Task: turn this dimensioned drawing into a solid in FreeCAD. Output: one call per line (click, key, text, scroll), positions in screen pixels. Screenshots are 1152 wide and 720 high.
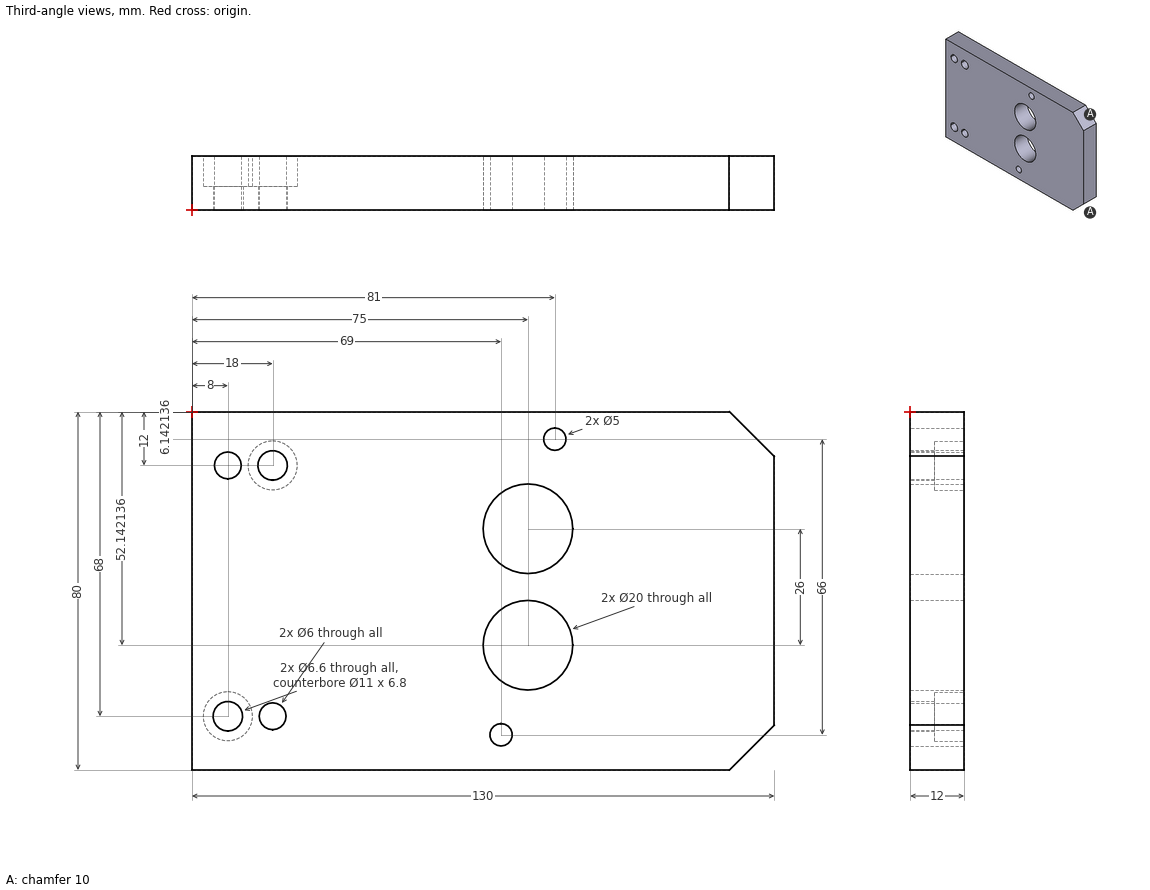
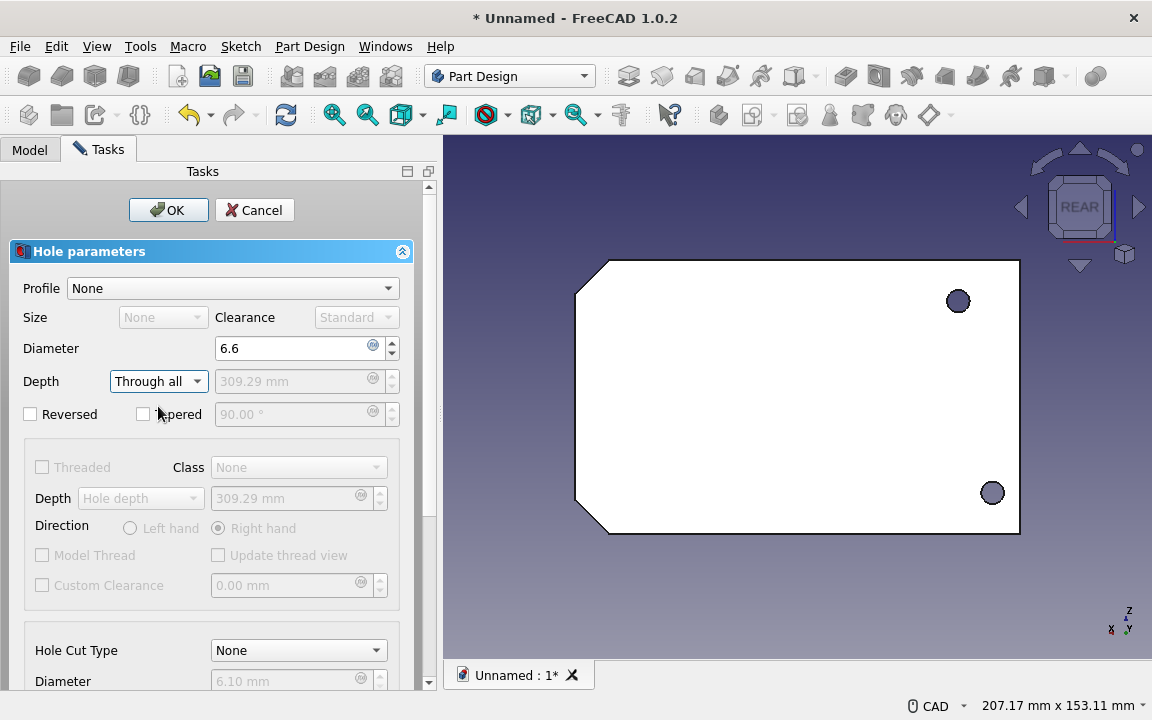
click(300, 650)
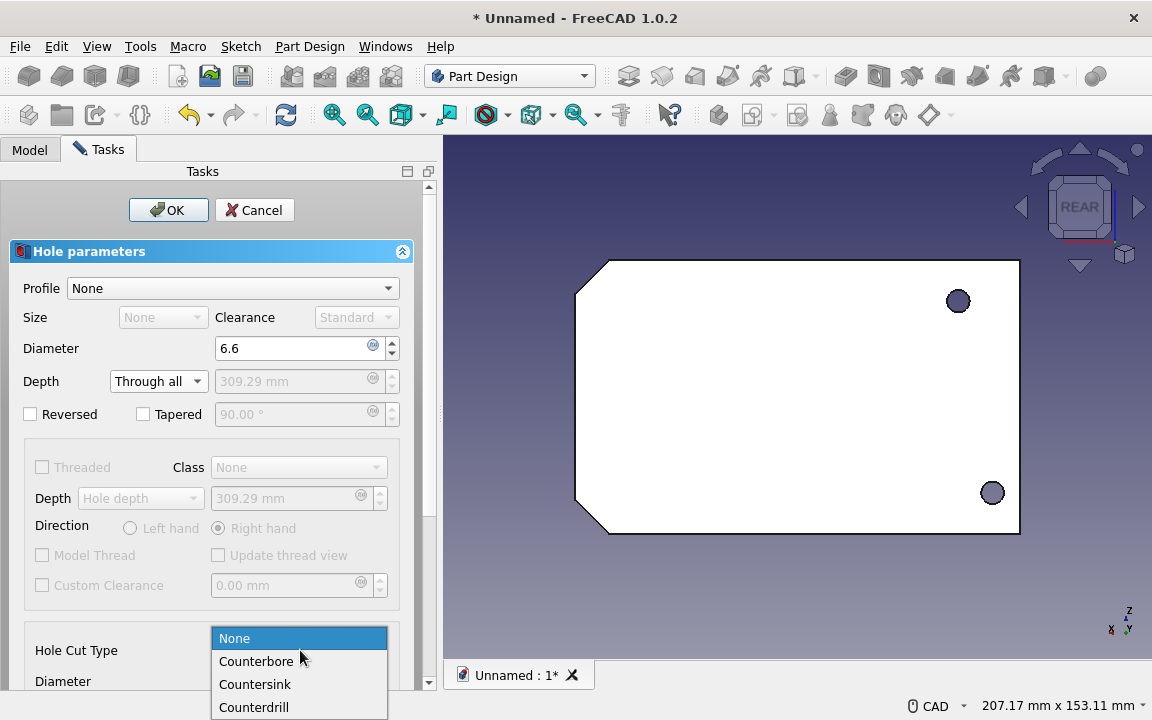
click(298, 662)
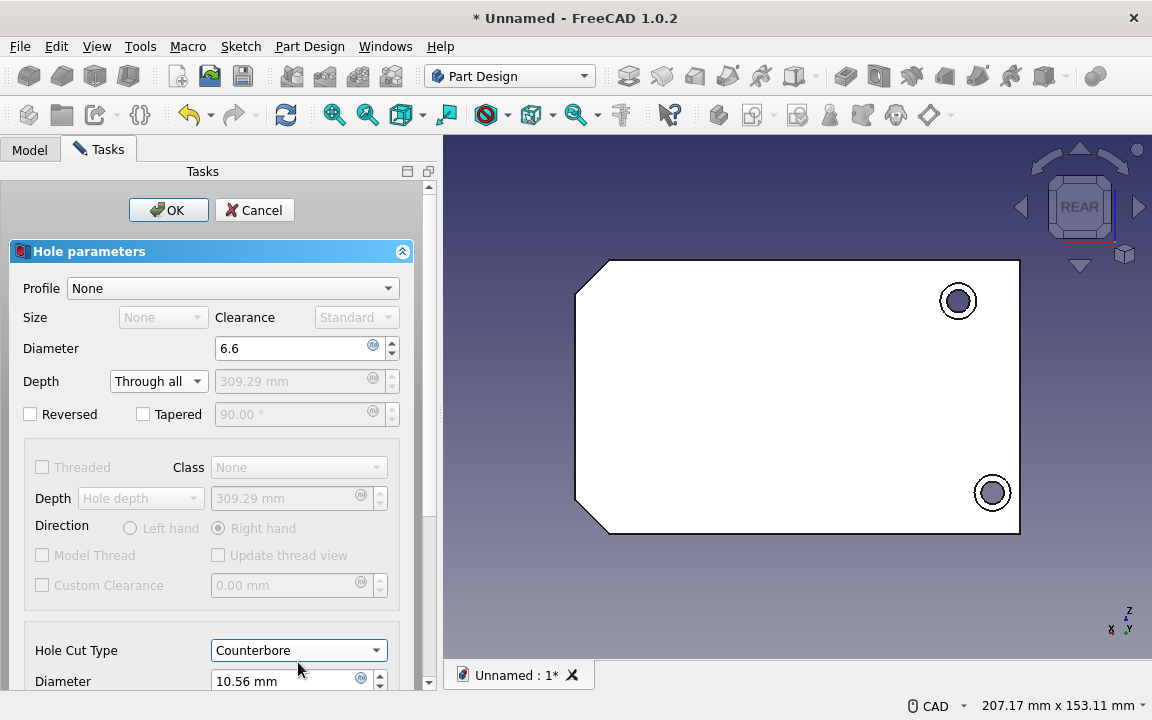
scroll(429, 436, down, 2)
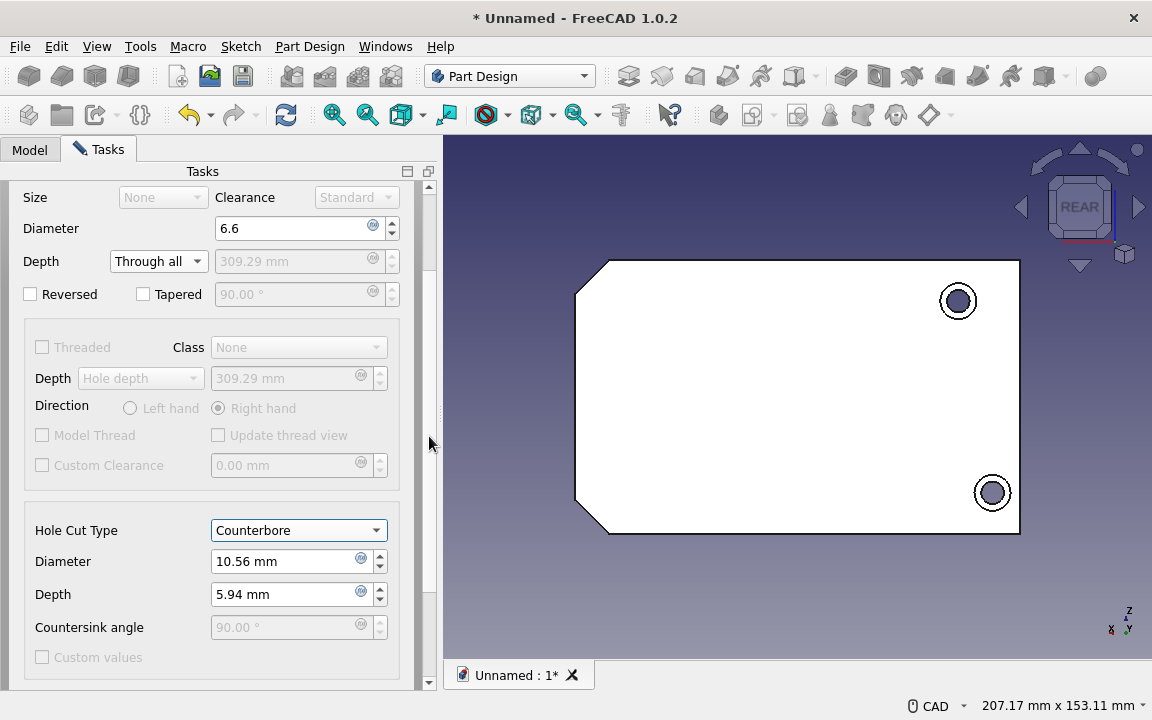
triple_click(292, 562)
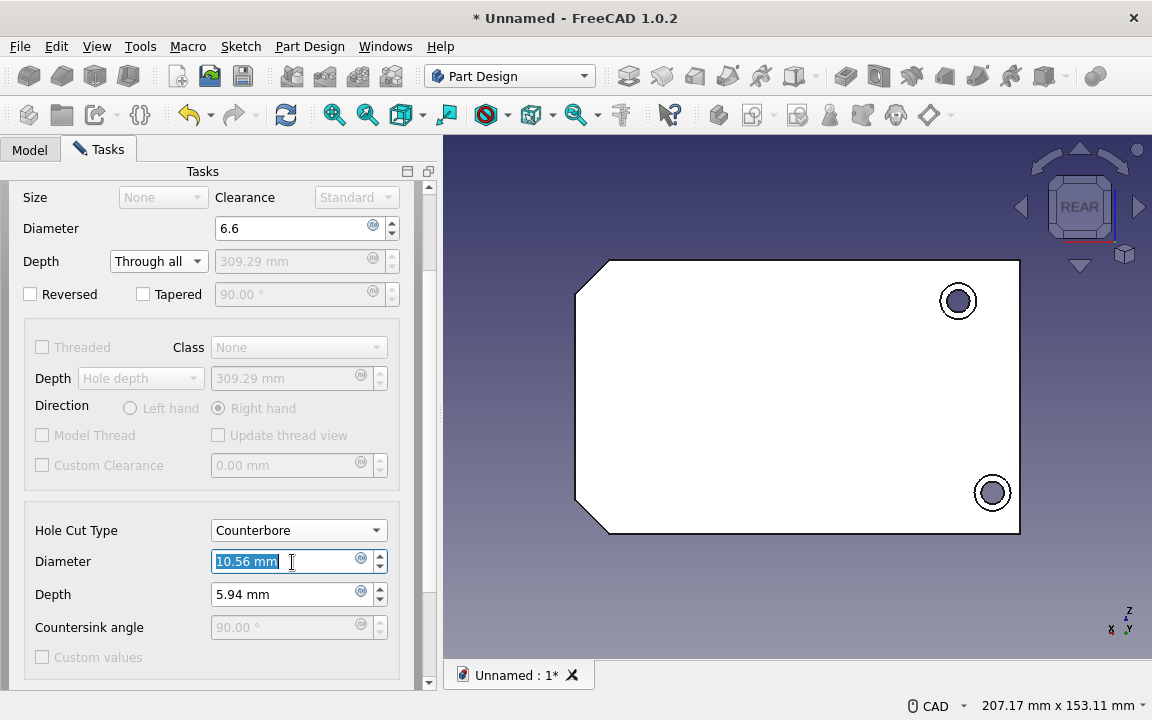
text(11)
key(Tab)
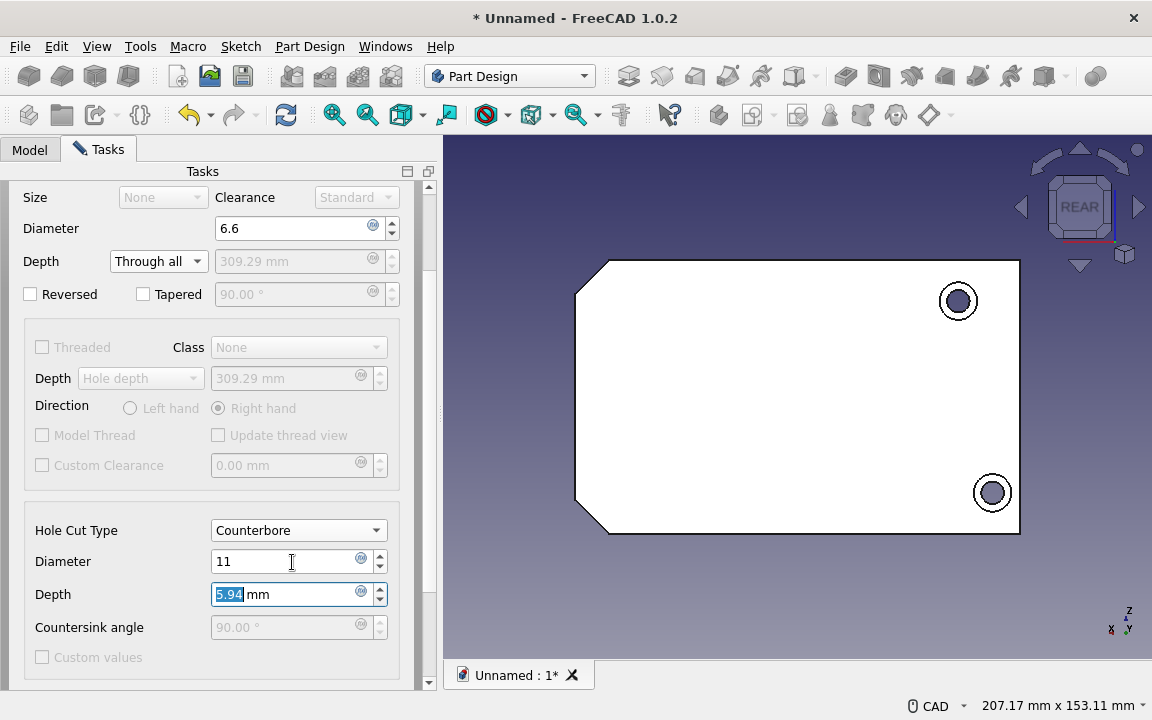
text(6.8)
key(Tab)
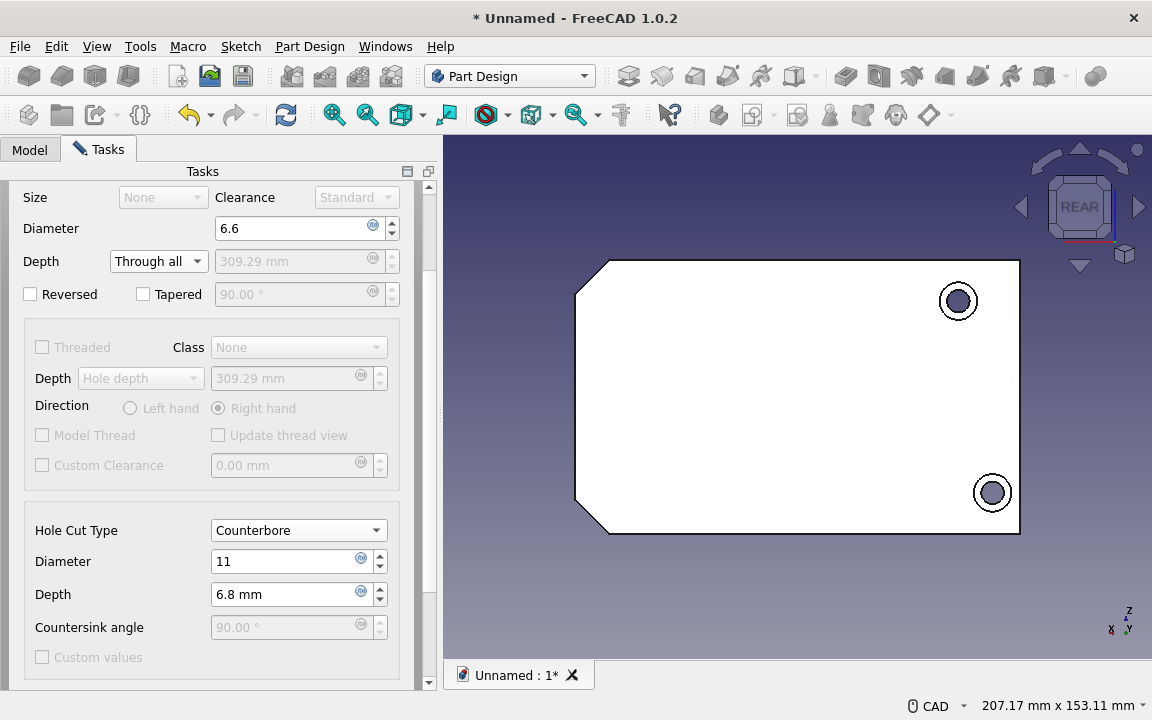
scroll(429, 436, up, 3)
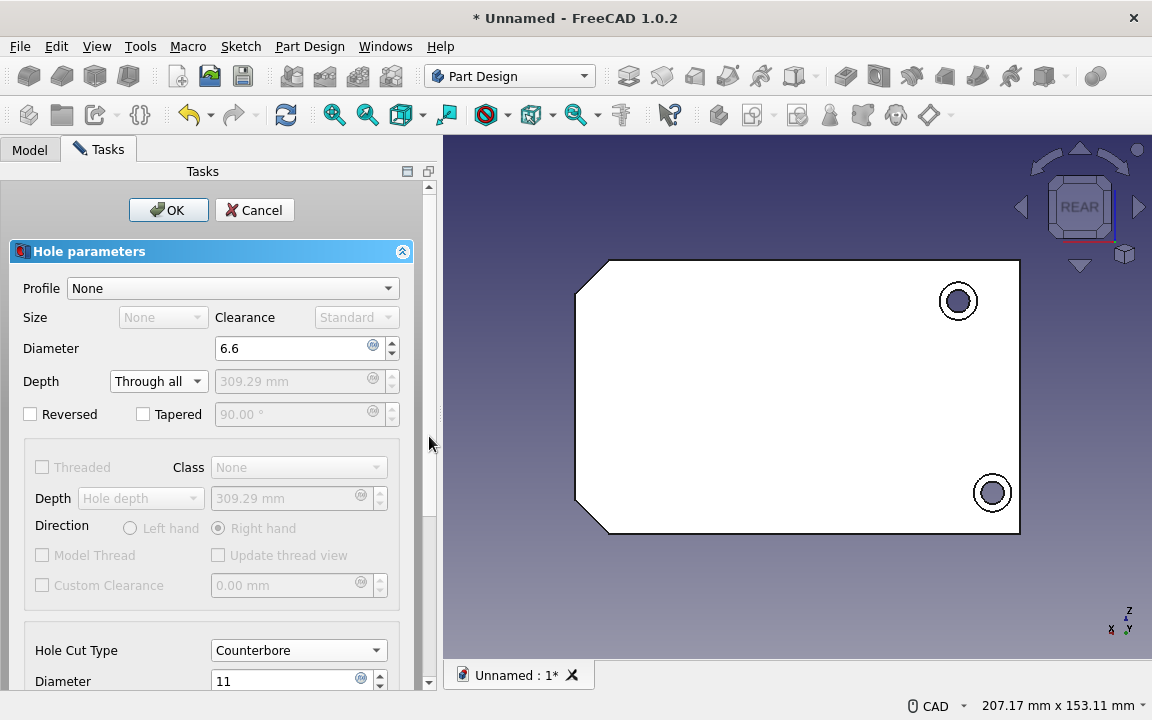
click(169, 210)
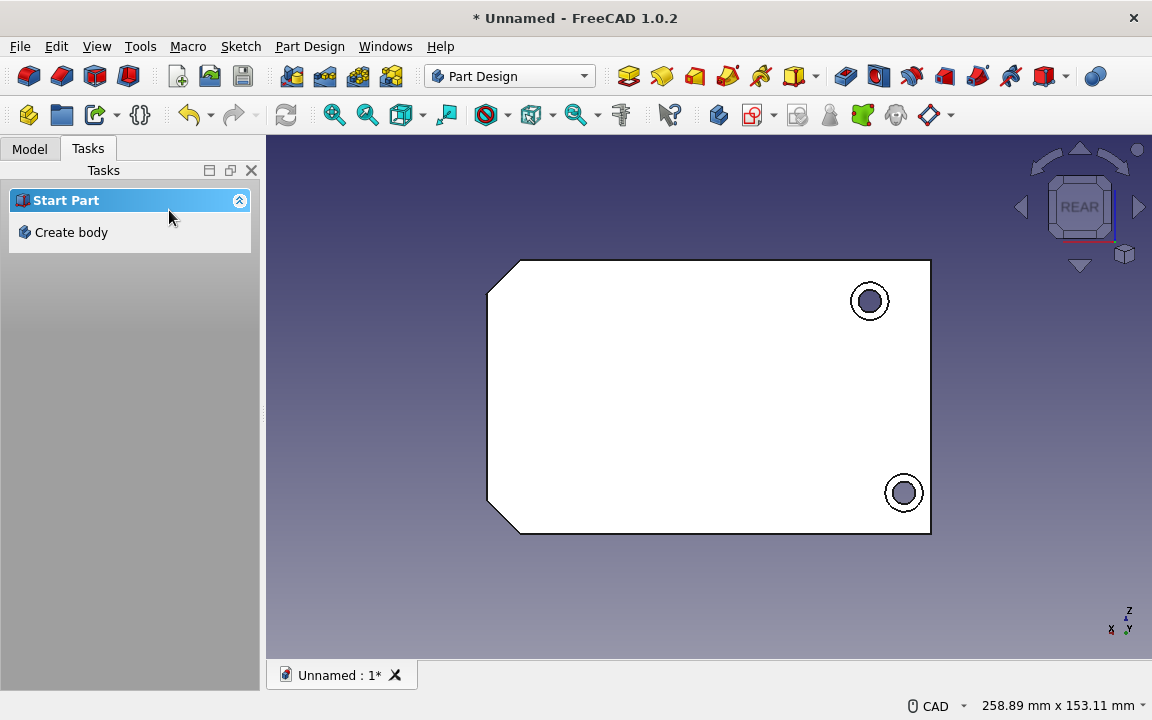
click(645, 396)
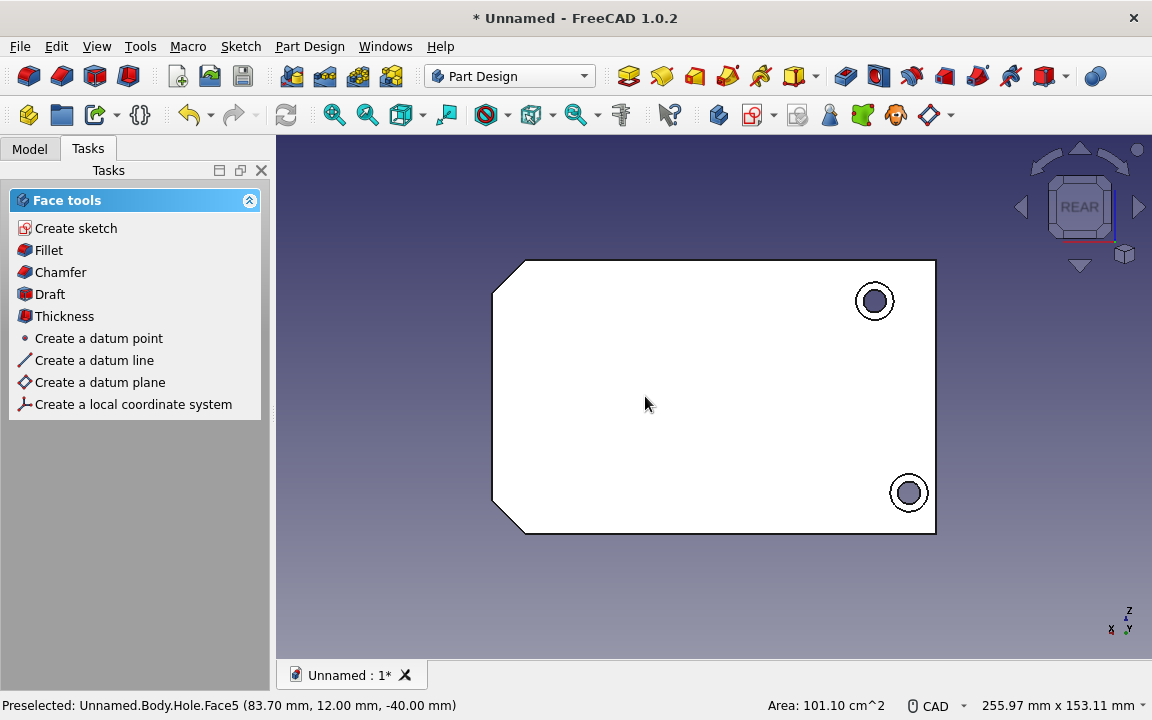
click(752, 116)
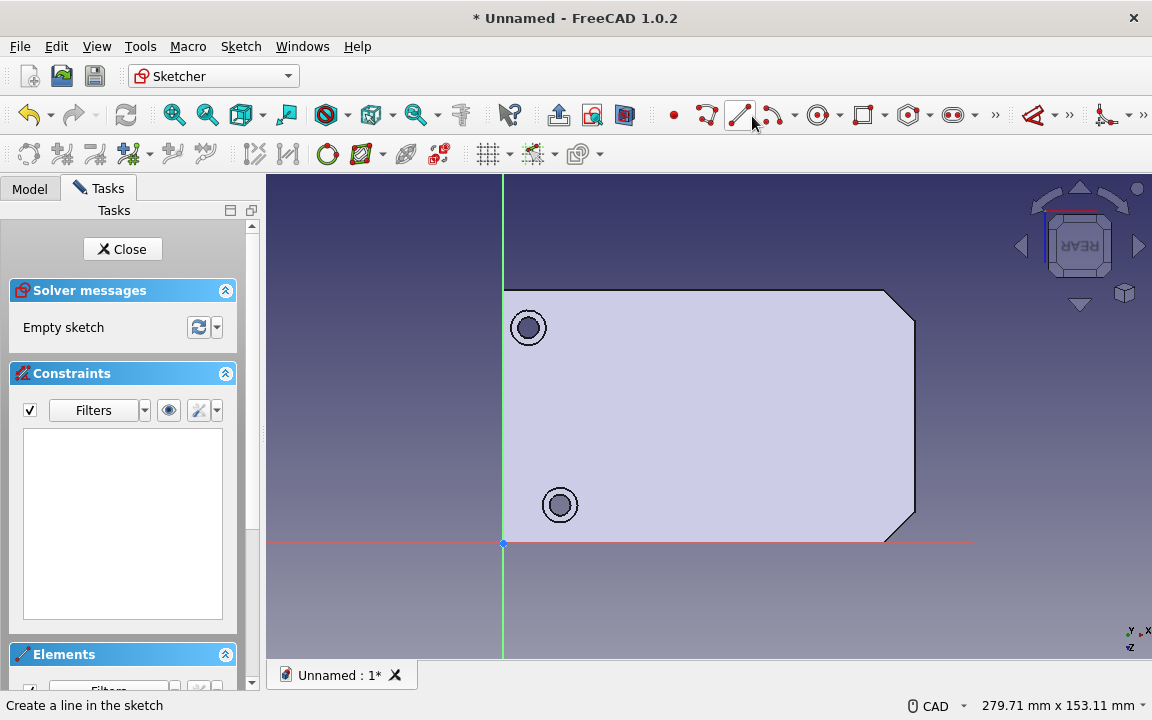
key(g)
key(c)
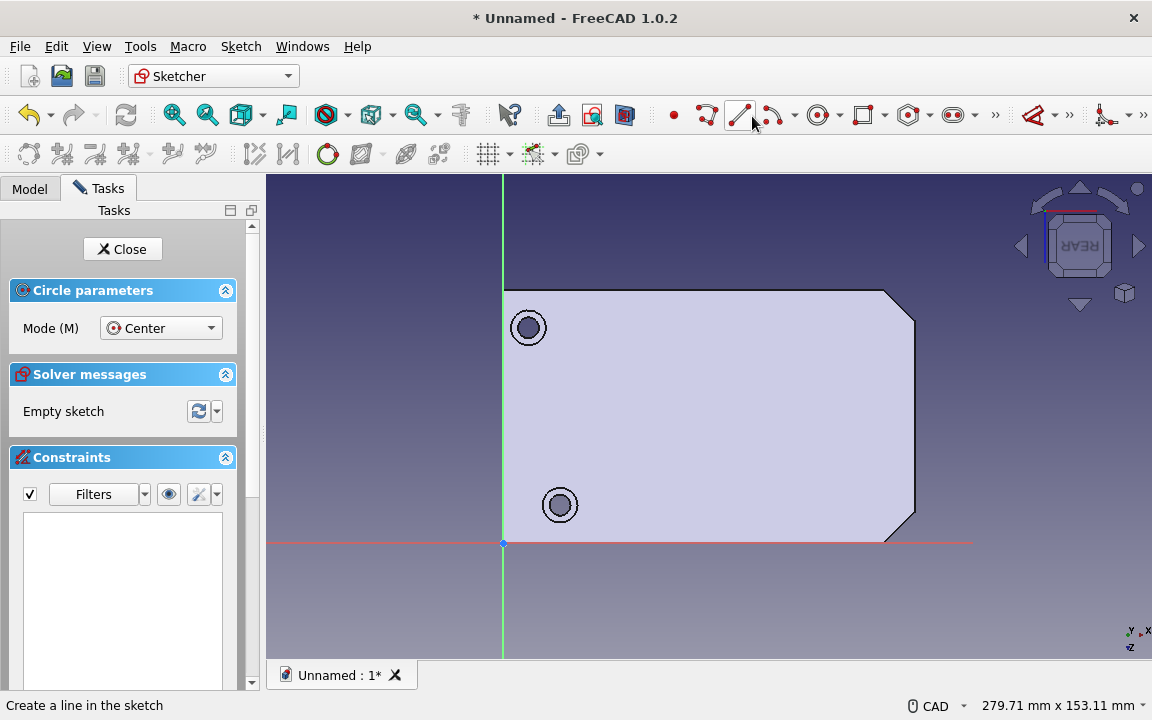
scroll(560, 328, up, 5)